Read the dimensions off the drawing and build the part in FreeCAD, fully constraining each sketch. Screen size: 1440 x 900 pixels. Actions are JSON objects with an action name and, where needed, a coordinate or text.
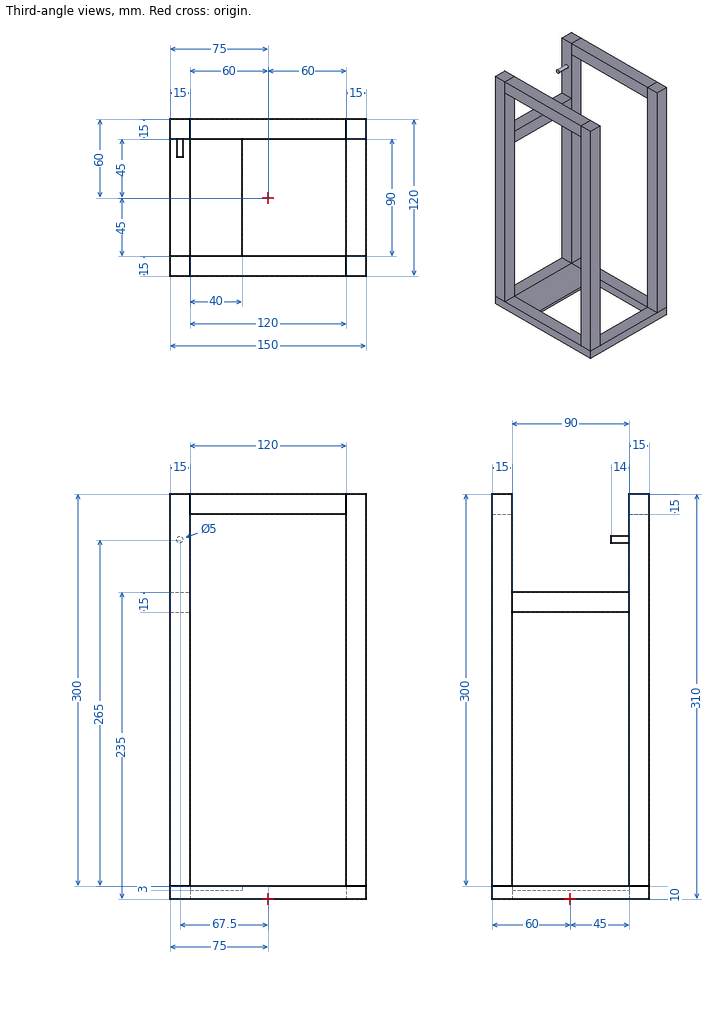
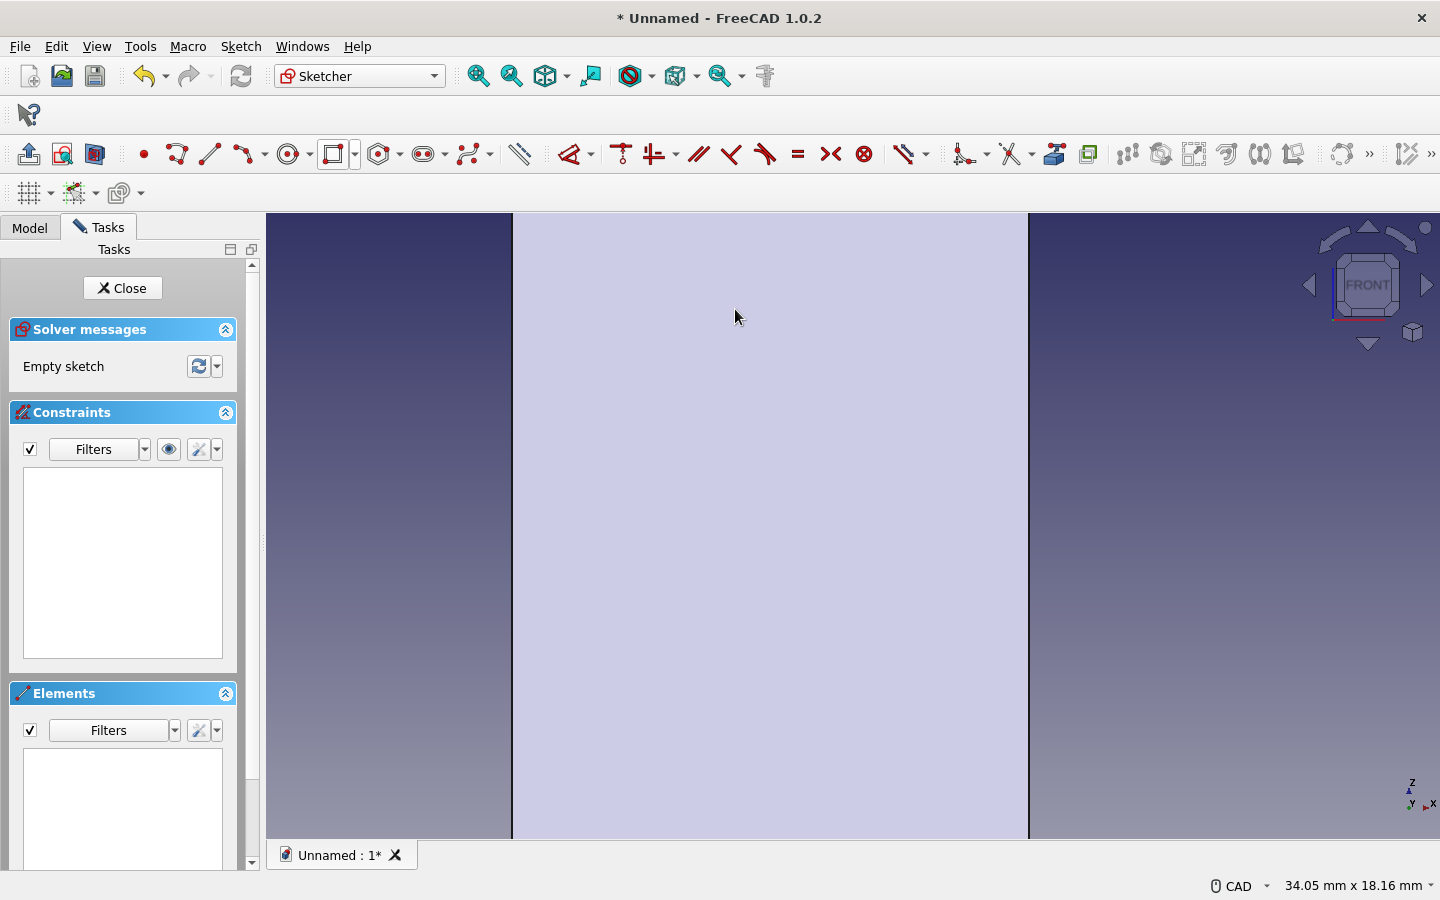
{"action": "scroll", "coordinate": [759, 528], "scroll_direction": "up", "scroll_amount": 4}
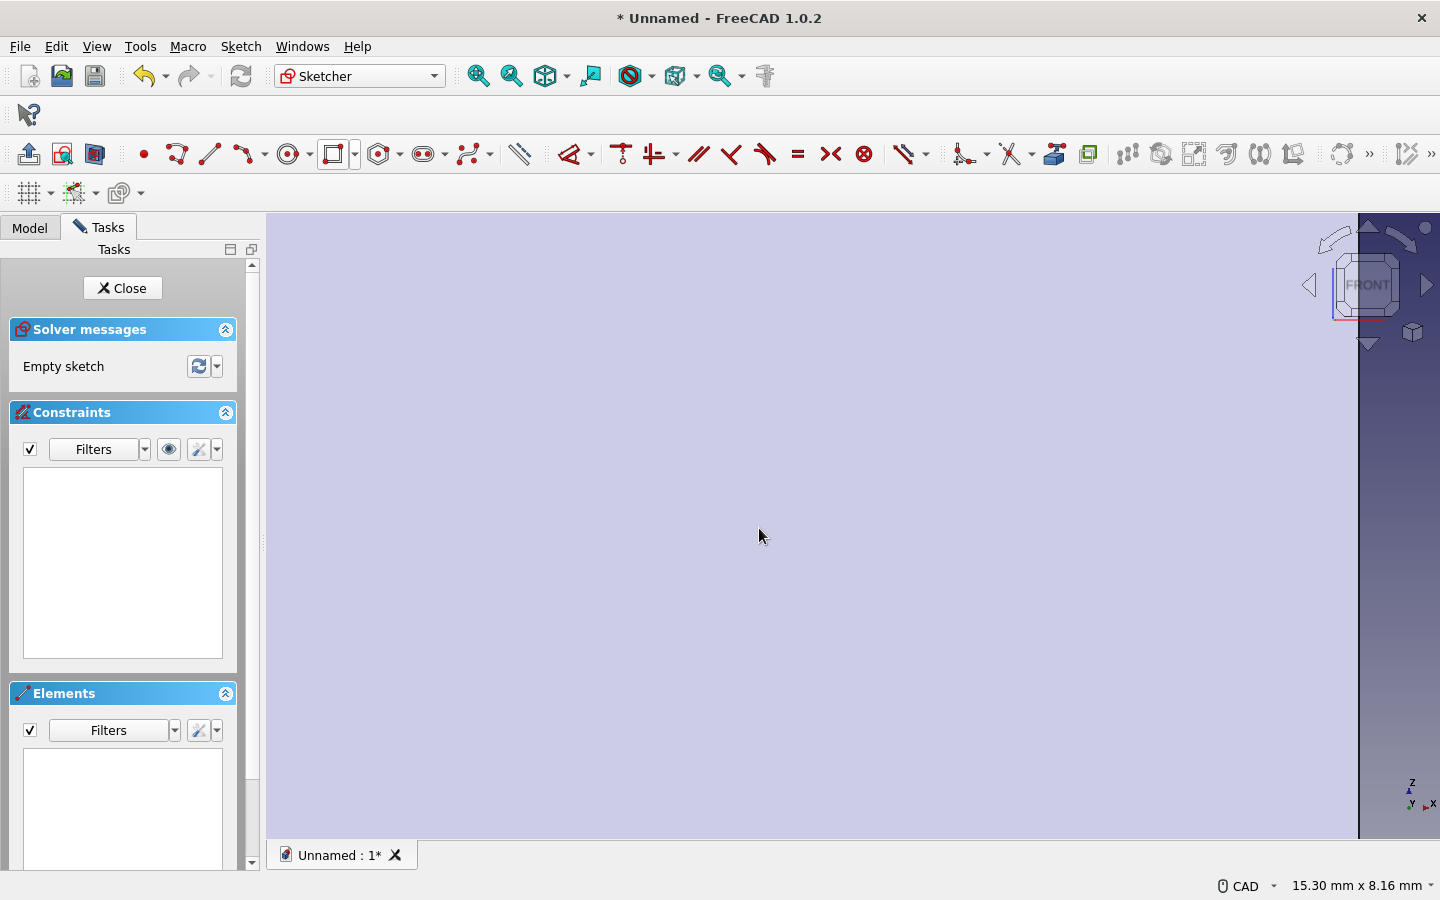
{"action": "left_click", "coordinate": [288, 154]}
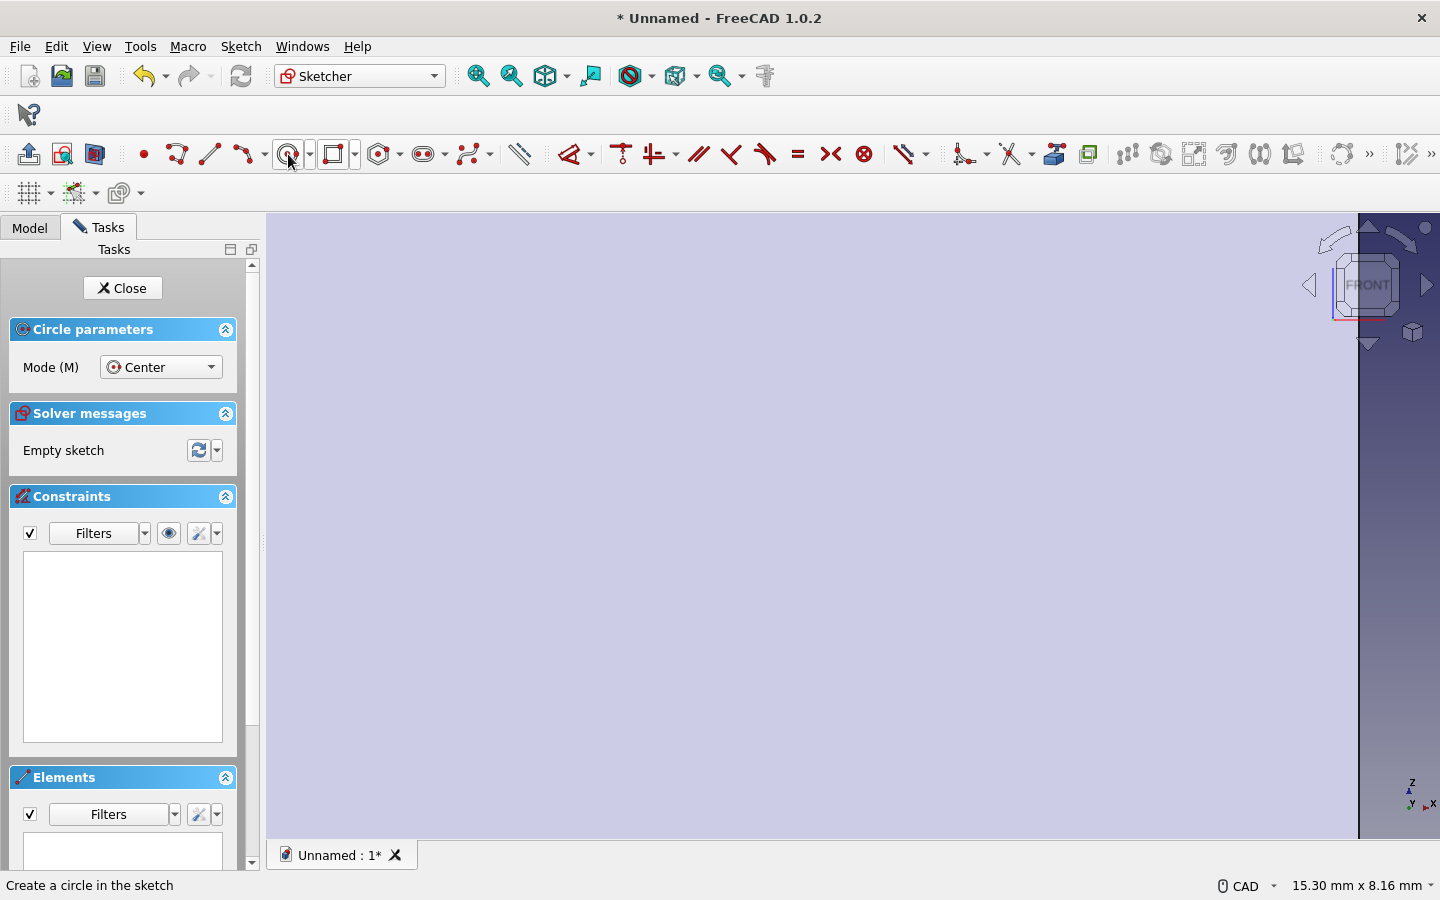
{"action": "left_click", "coordinate": [784, 526]}
{"action": "left_click", "coordinate": [919, 390]}
{"action": "key", "text": "Escape"}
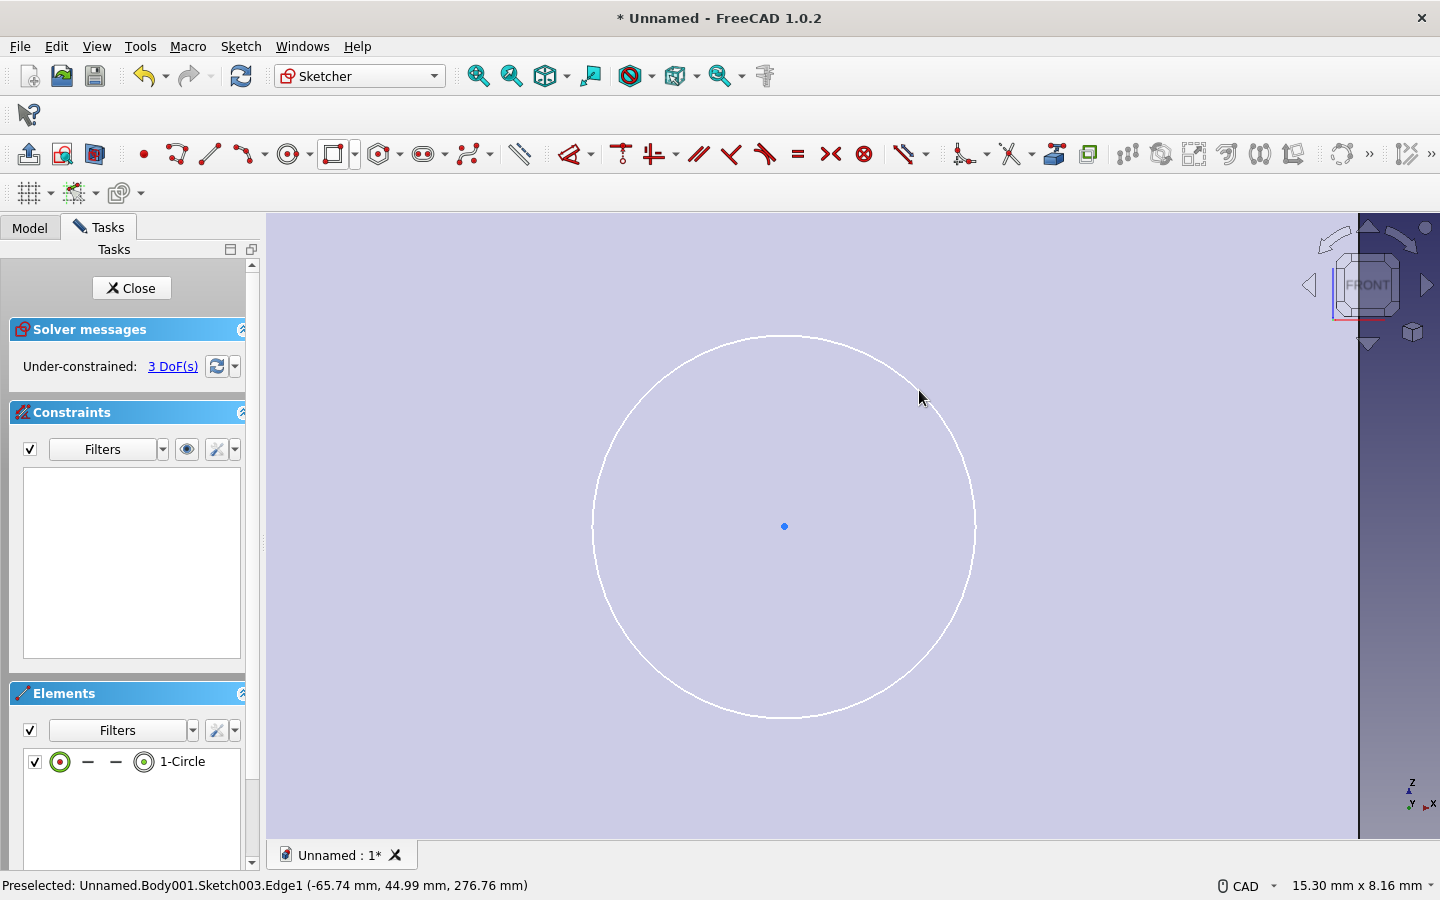
{"action": "left_click", "coordinate": [568, 154]}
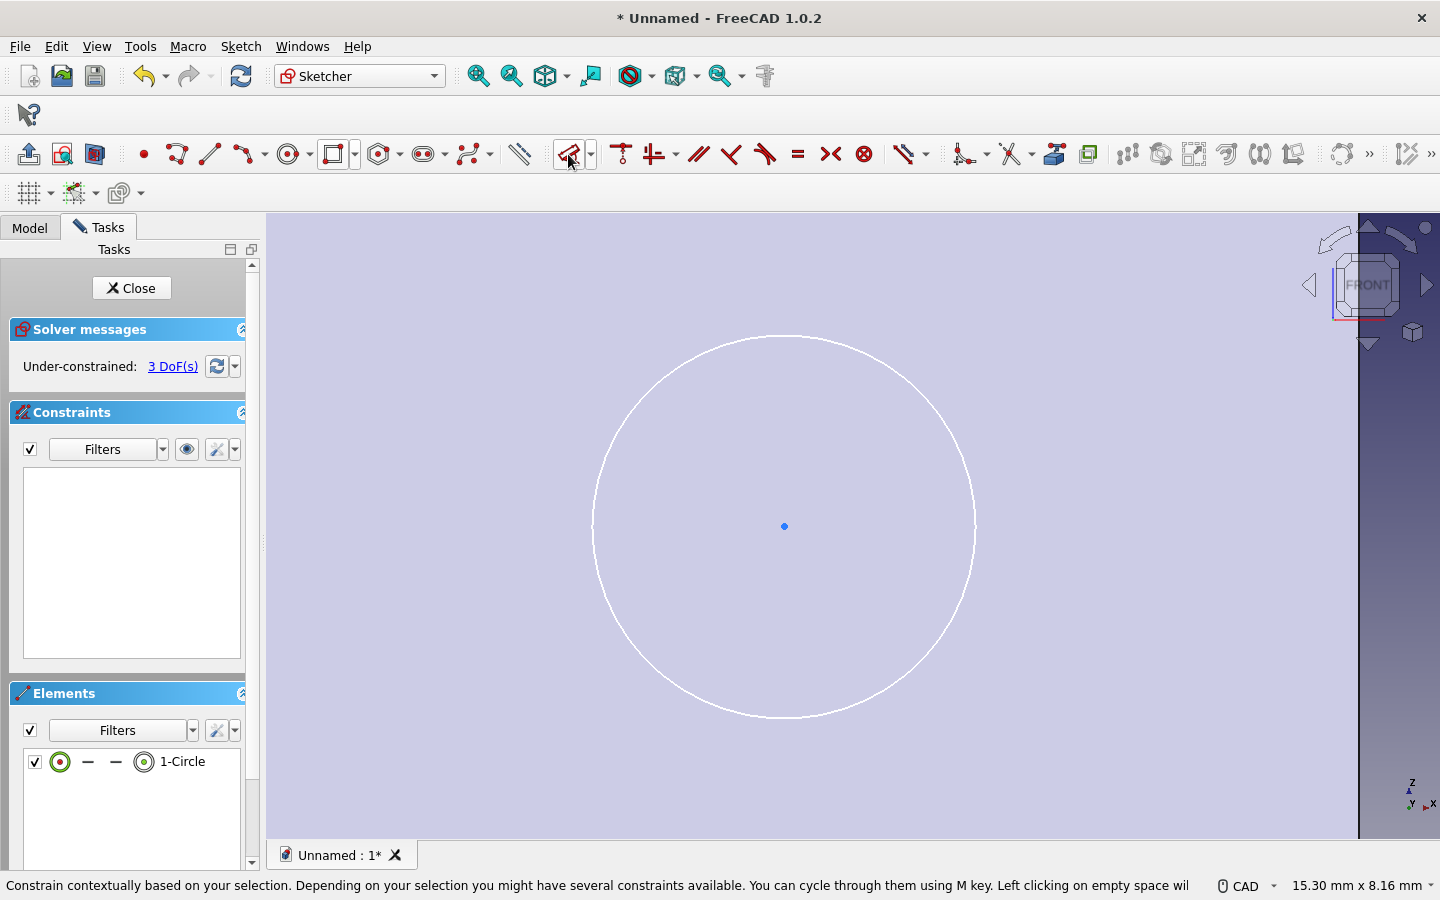
{"action": "left_click", "coordinate": [919, 391]}
{"action": "left_click", "coordinate": [942, 368]}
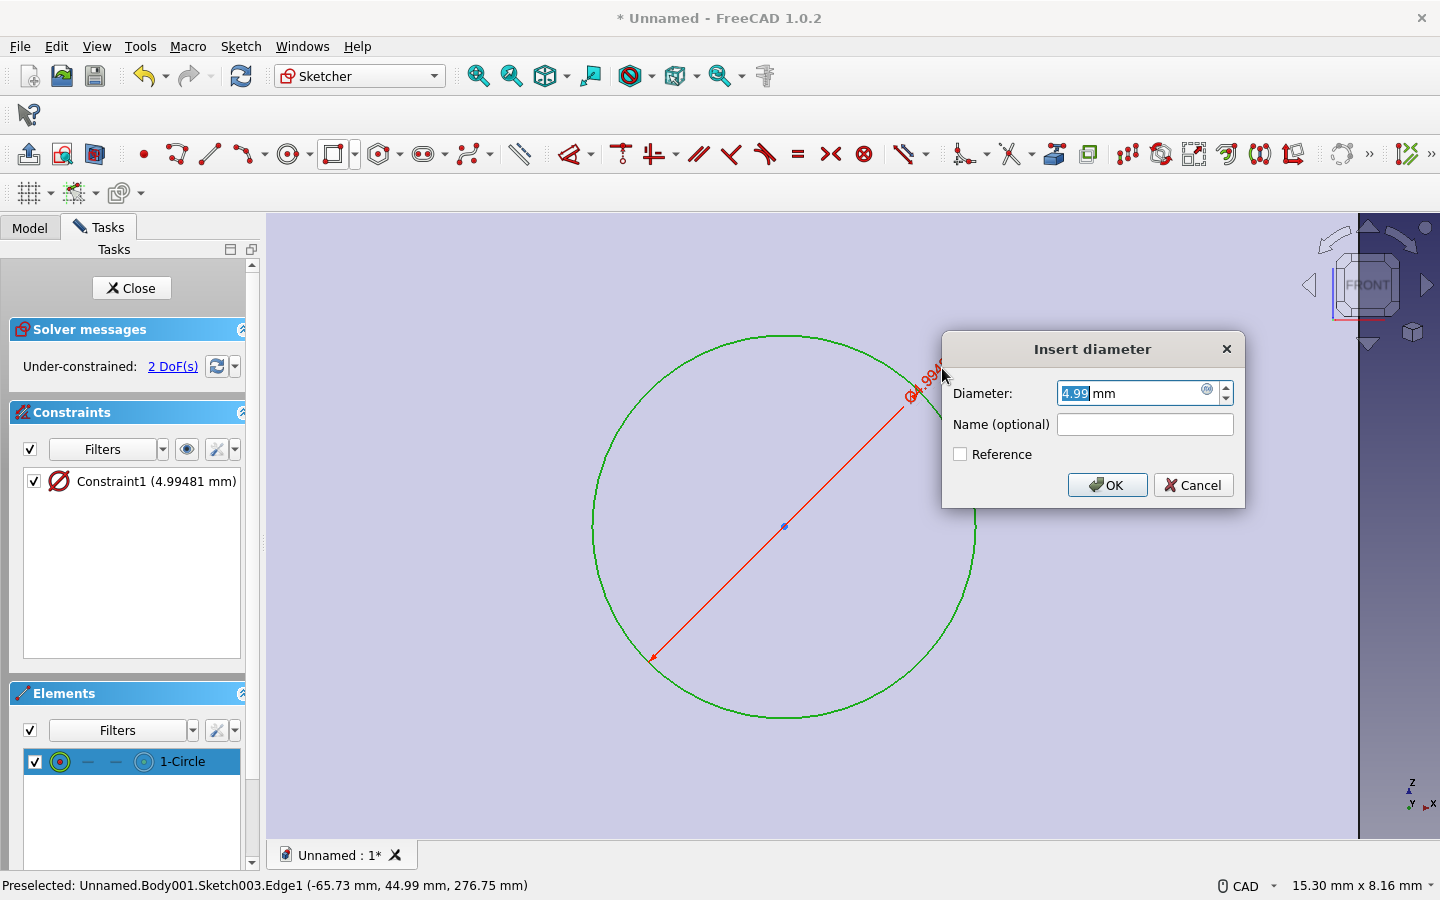
{"action": "type", "text": "5"}
{"action": "key", "text": "Return"}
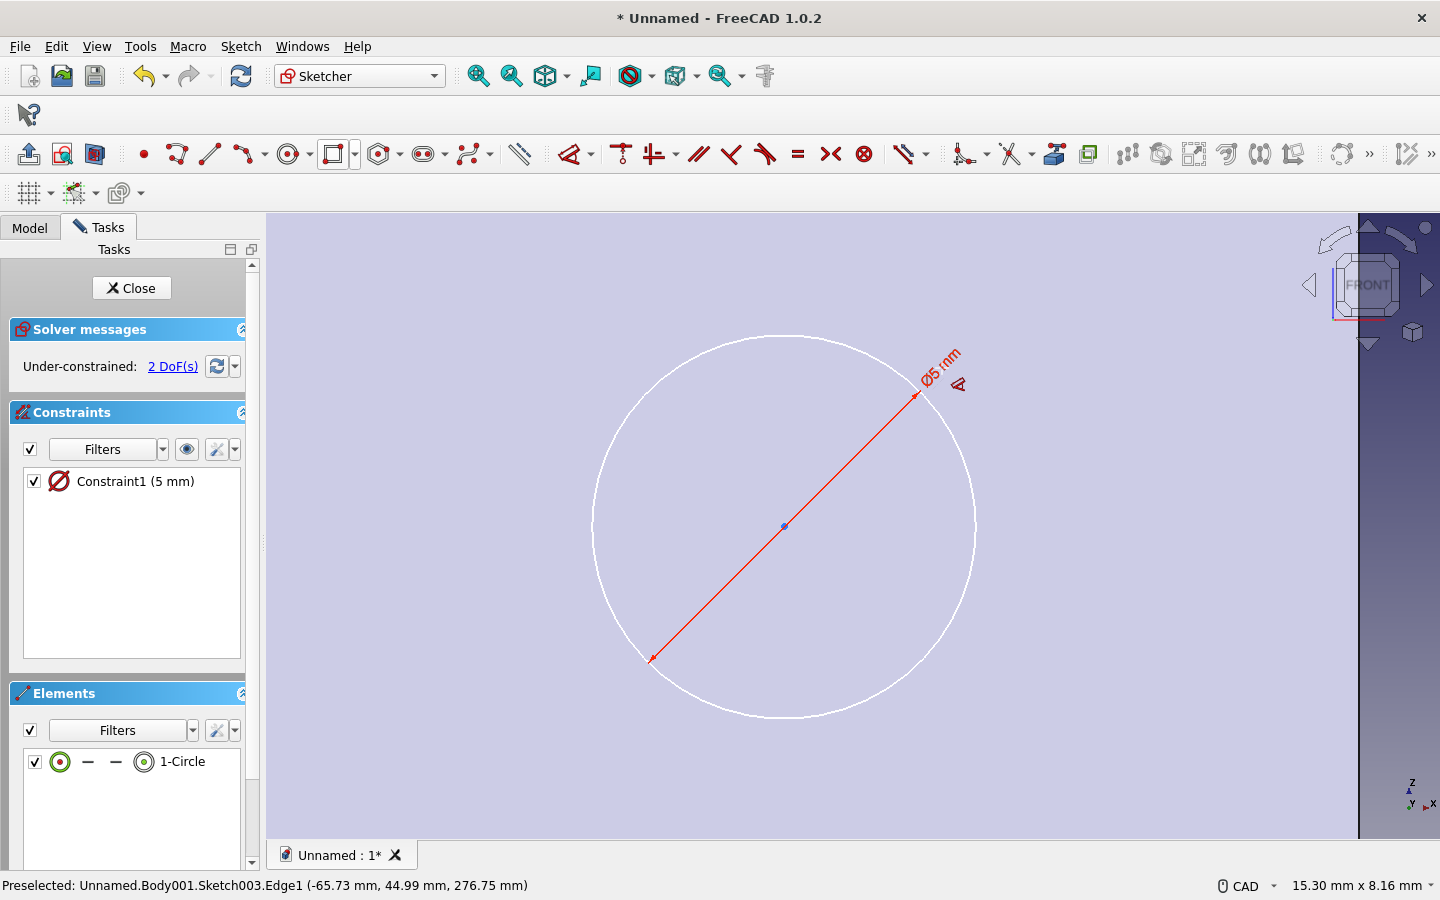
{"action": "left_click", "coordinate": [784, 527]}
{"action": "left_click", "coordinate": [750, 669]}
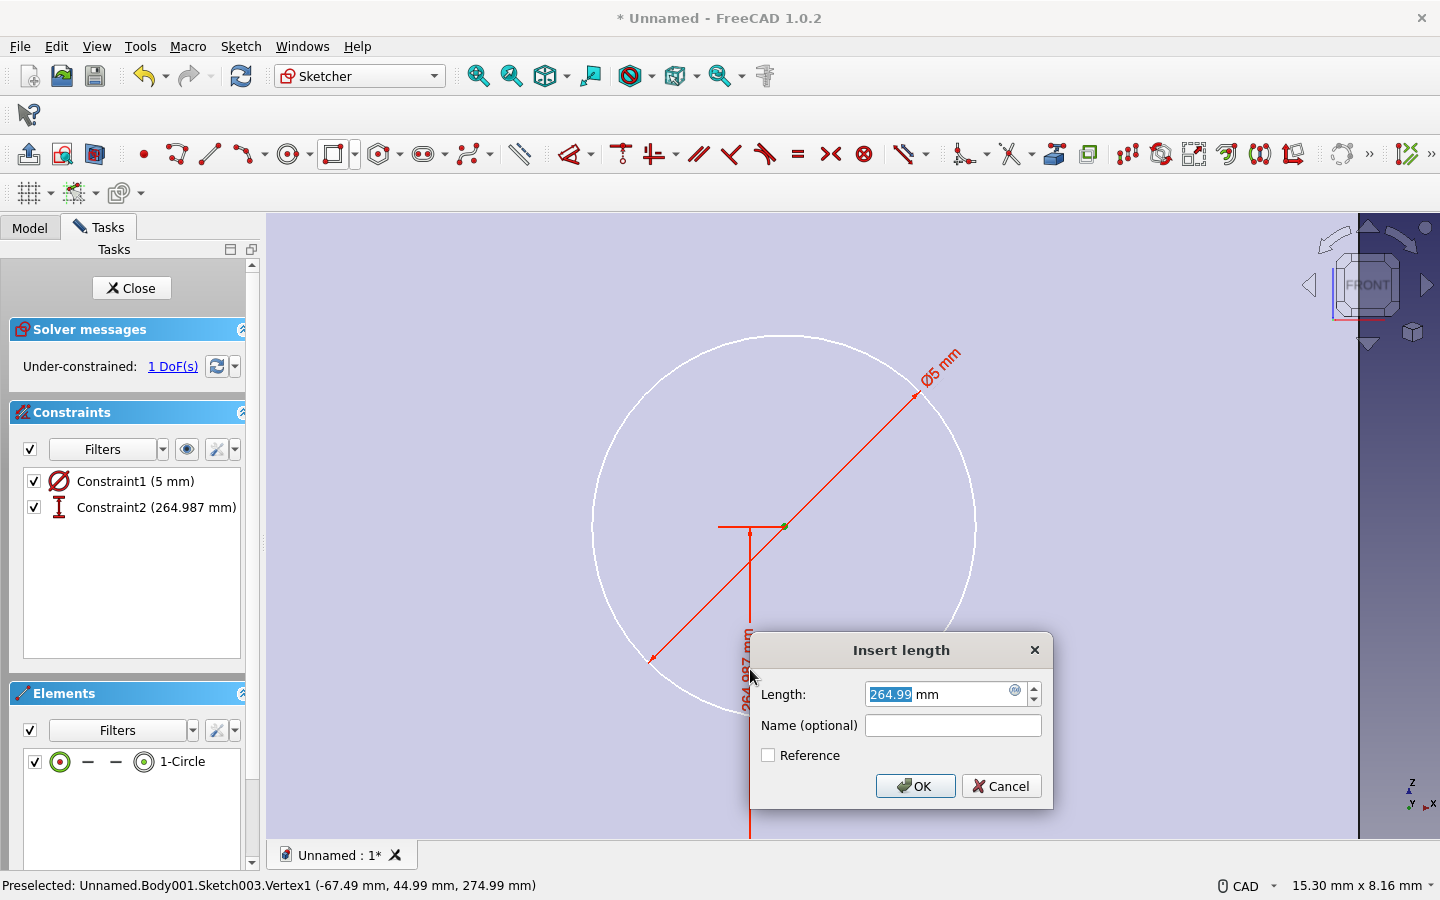
{"action": "type", "text": "265"}
{"action": "key", "text": "Return"}